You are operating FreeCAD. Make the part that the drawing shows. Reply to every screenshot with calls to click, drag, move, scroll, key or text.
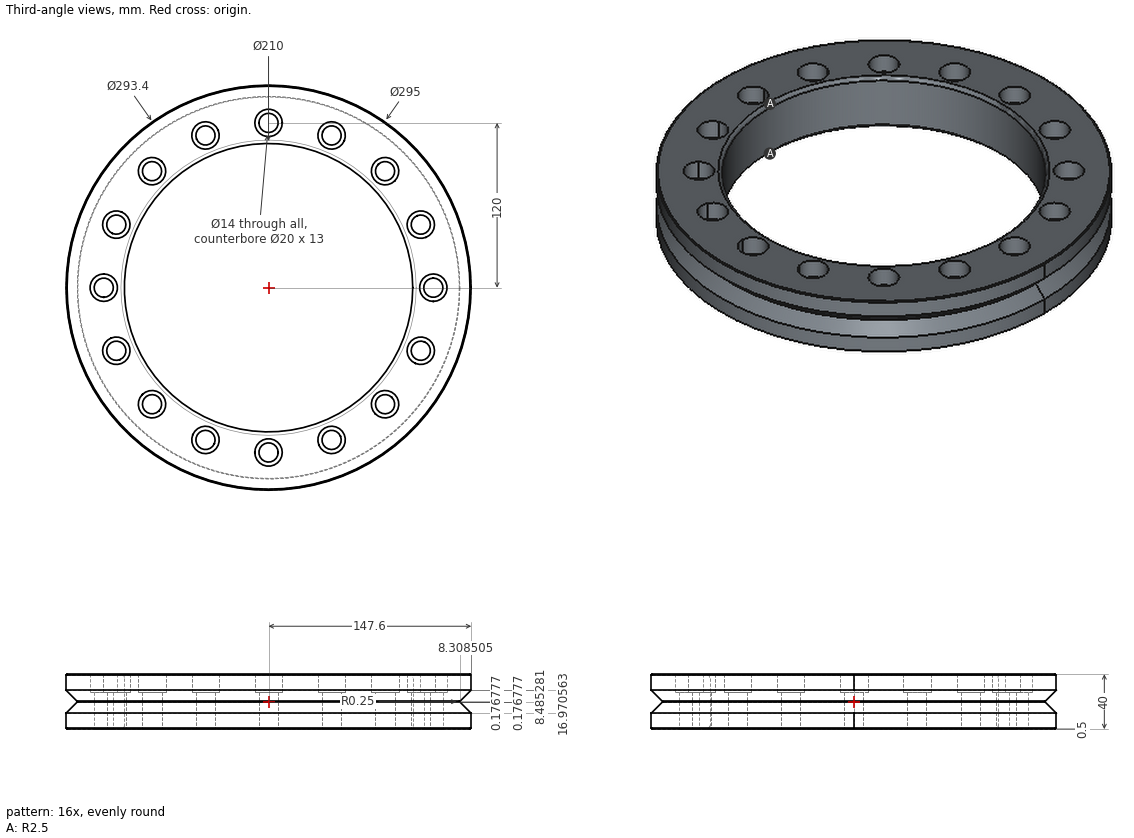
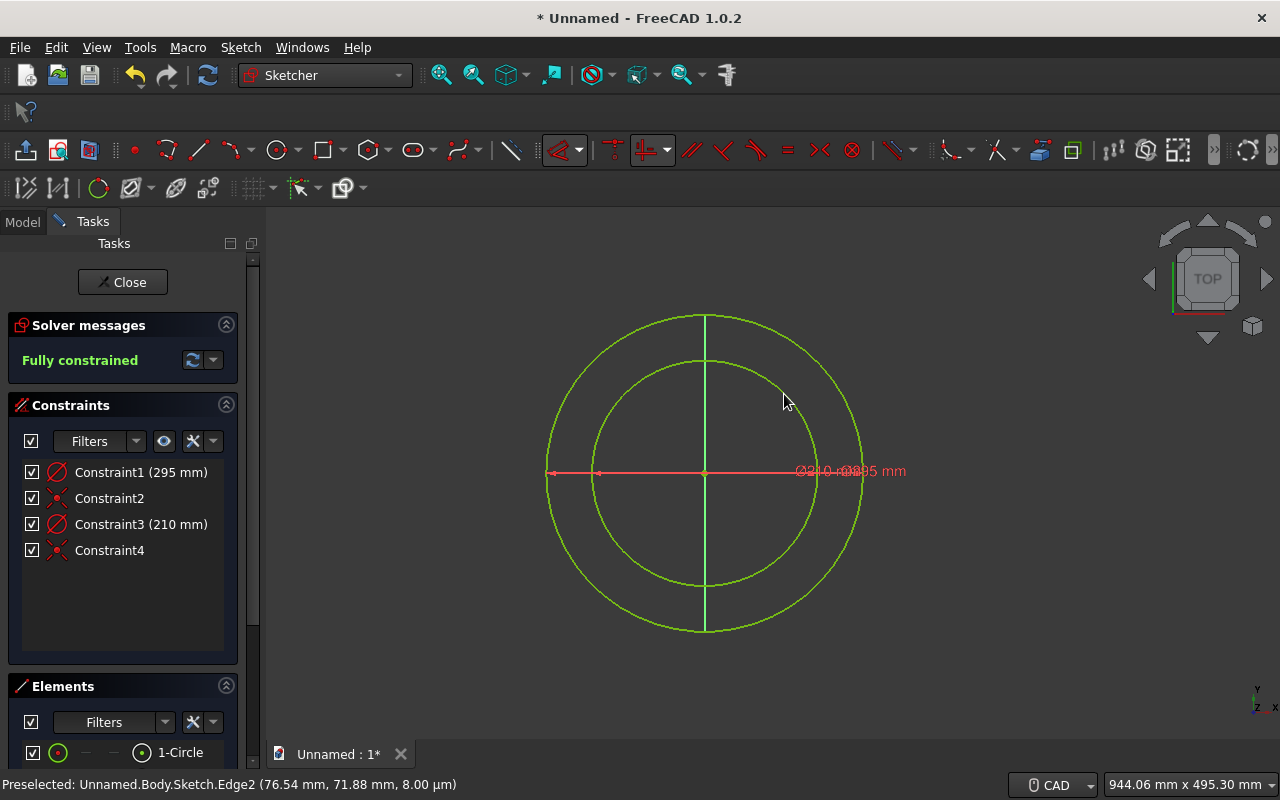
click(123, 282)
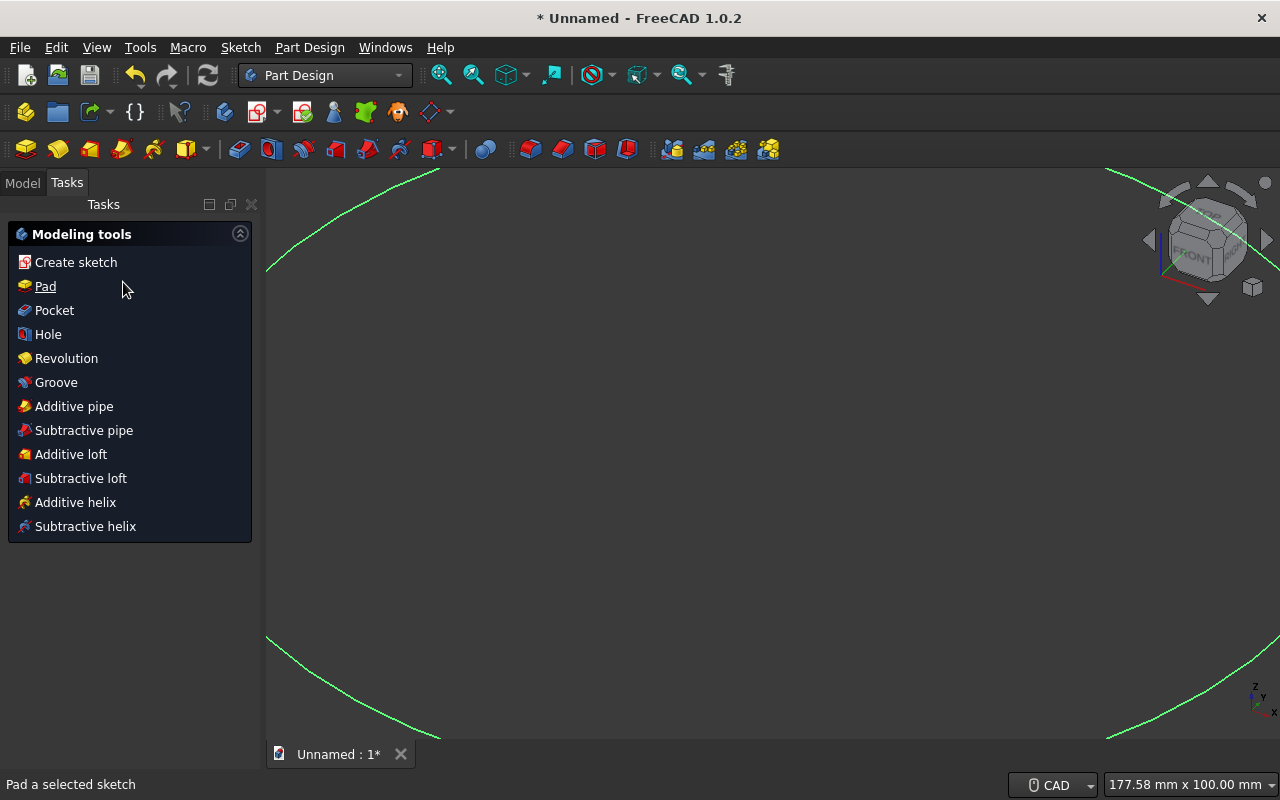
click(26, 150)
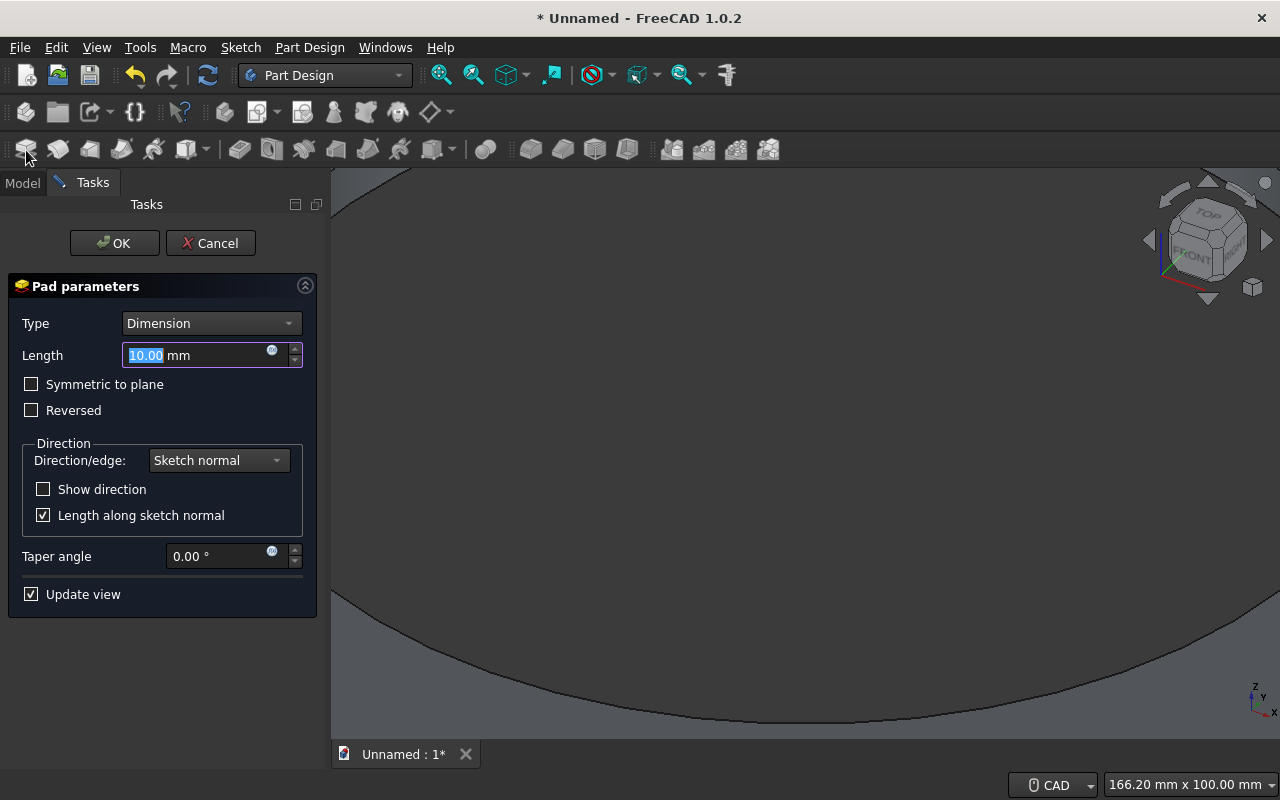
text(40)
key(Tab)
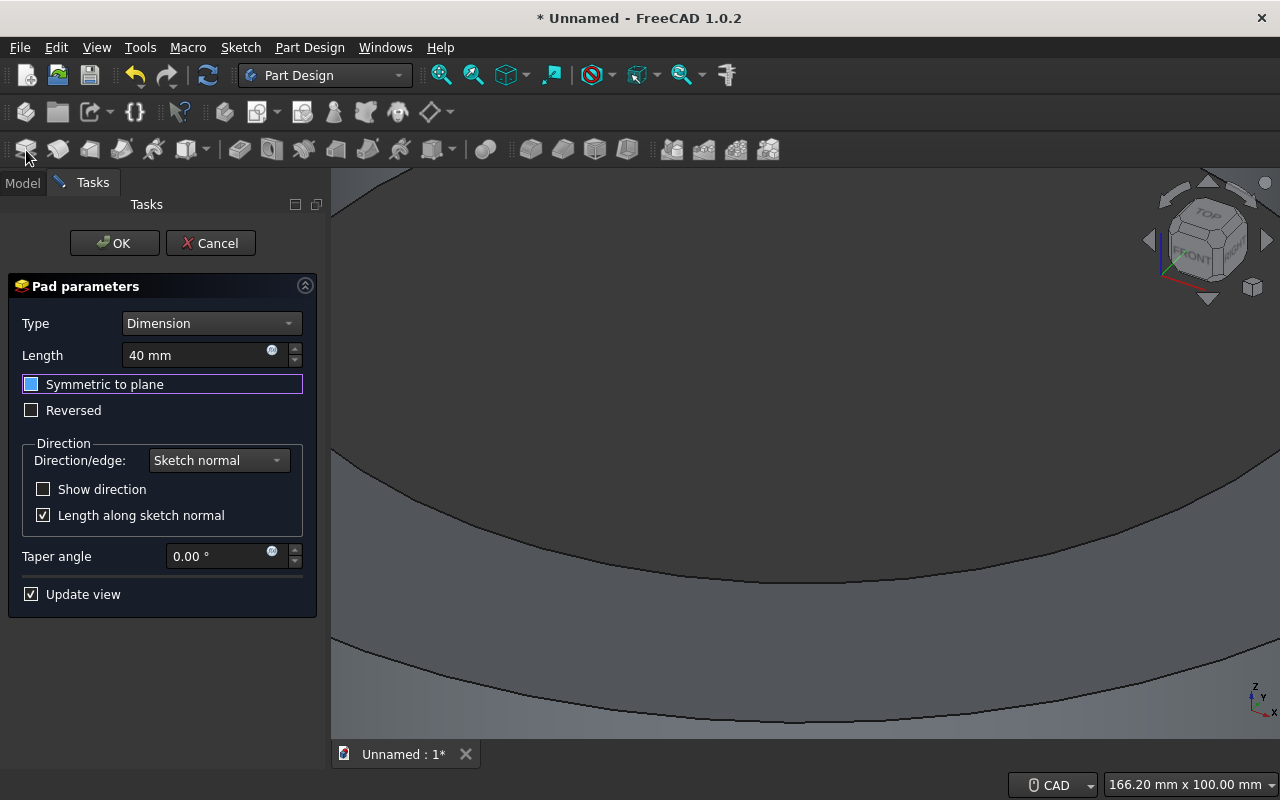
click(30, 384)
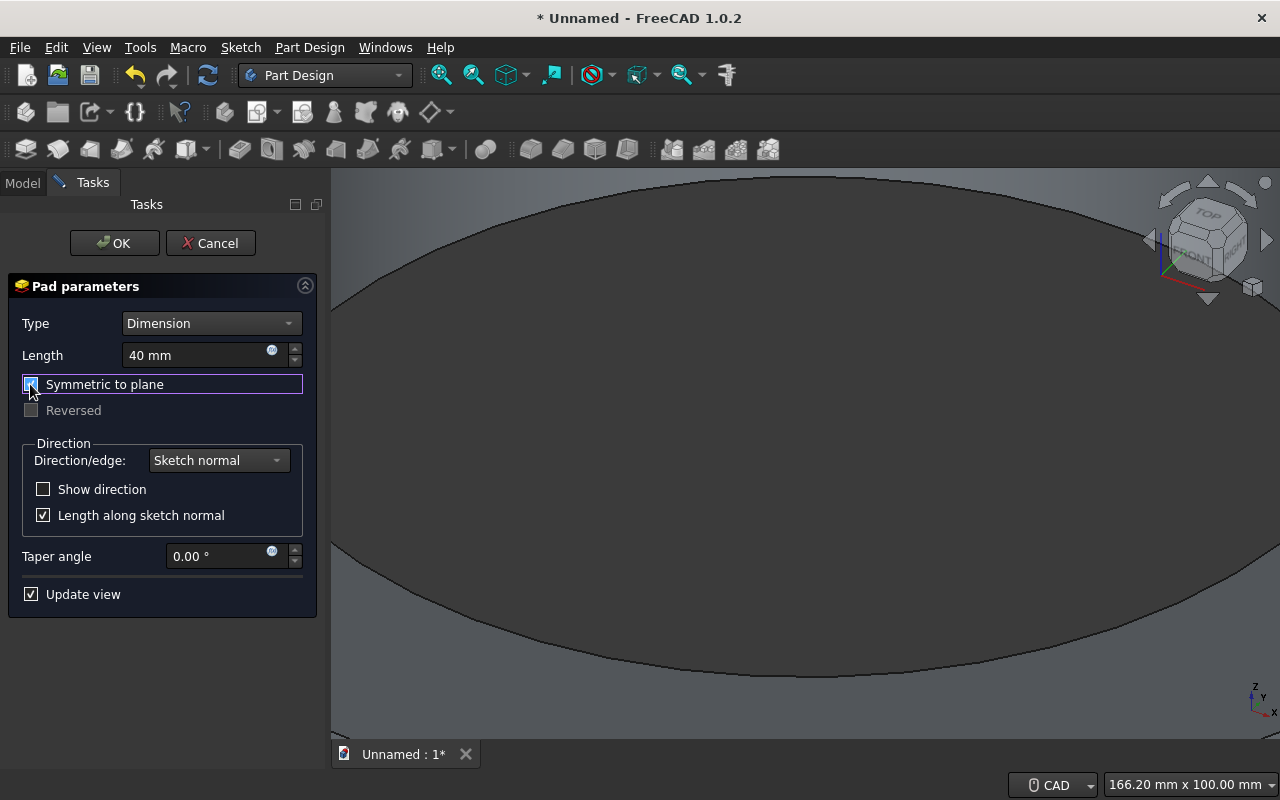
click(115, 243)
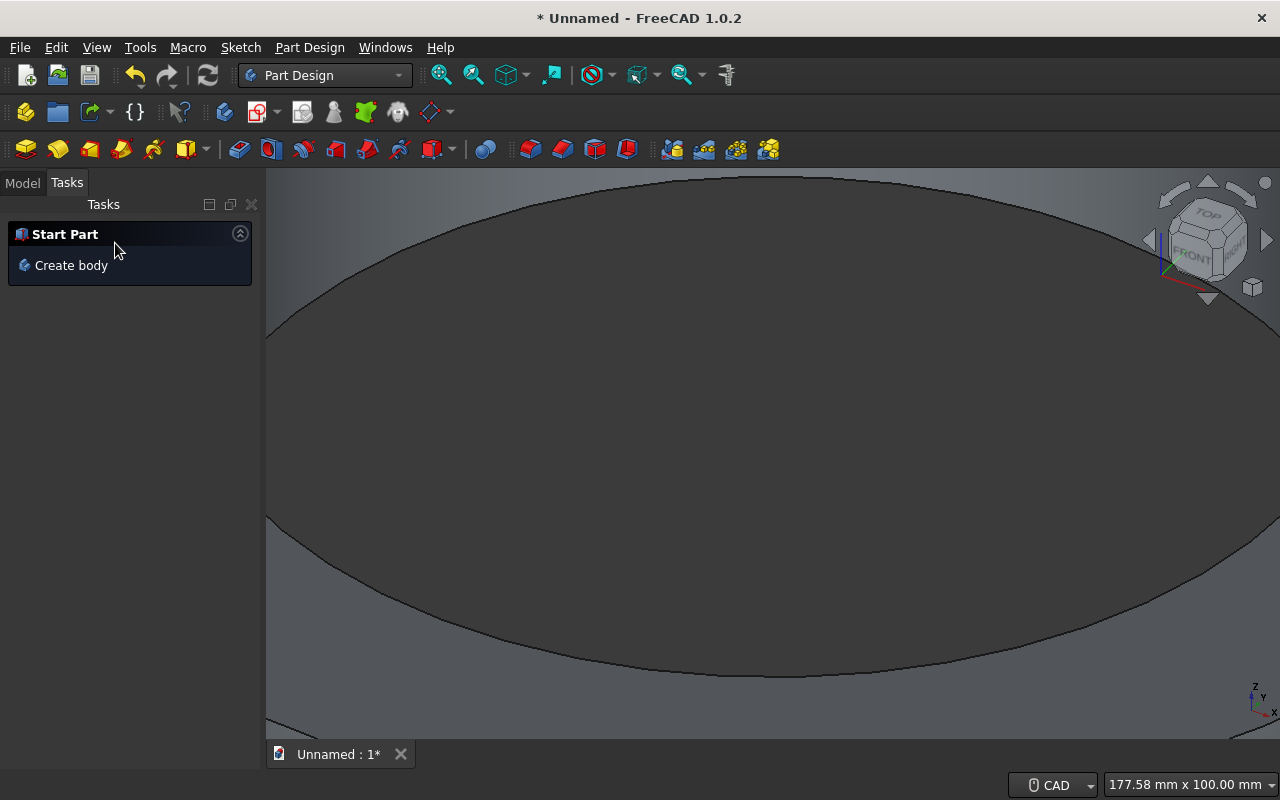
click(442, 76)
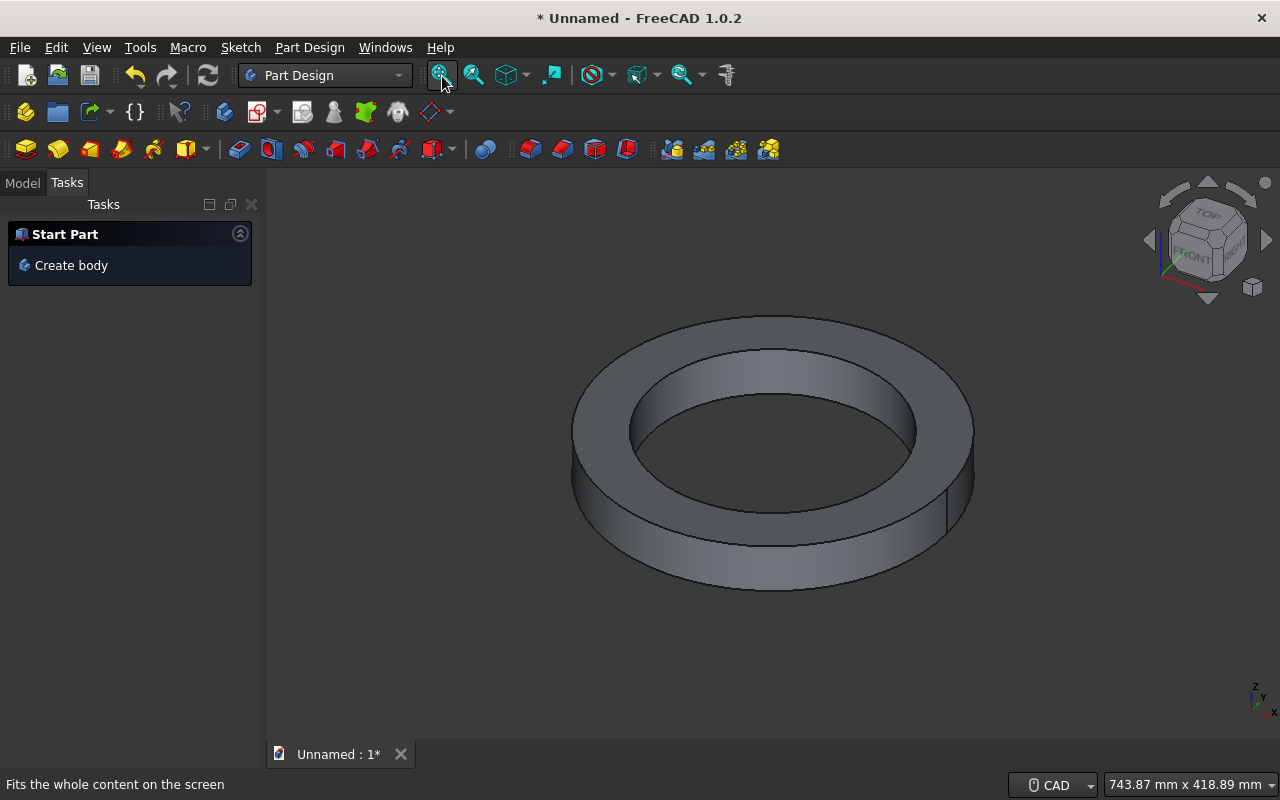
click(922, 480)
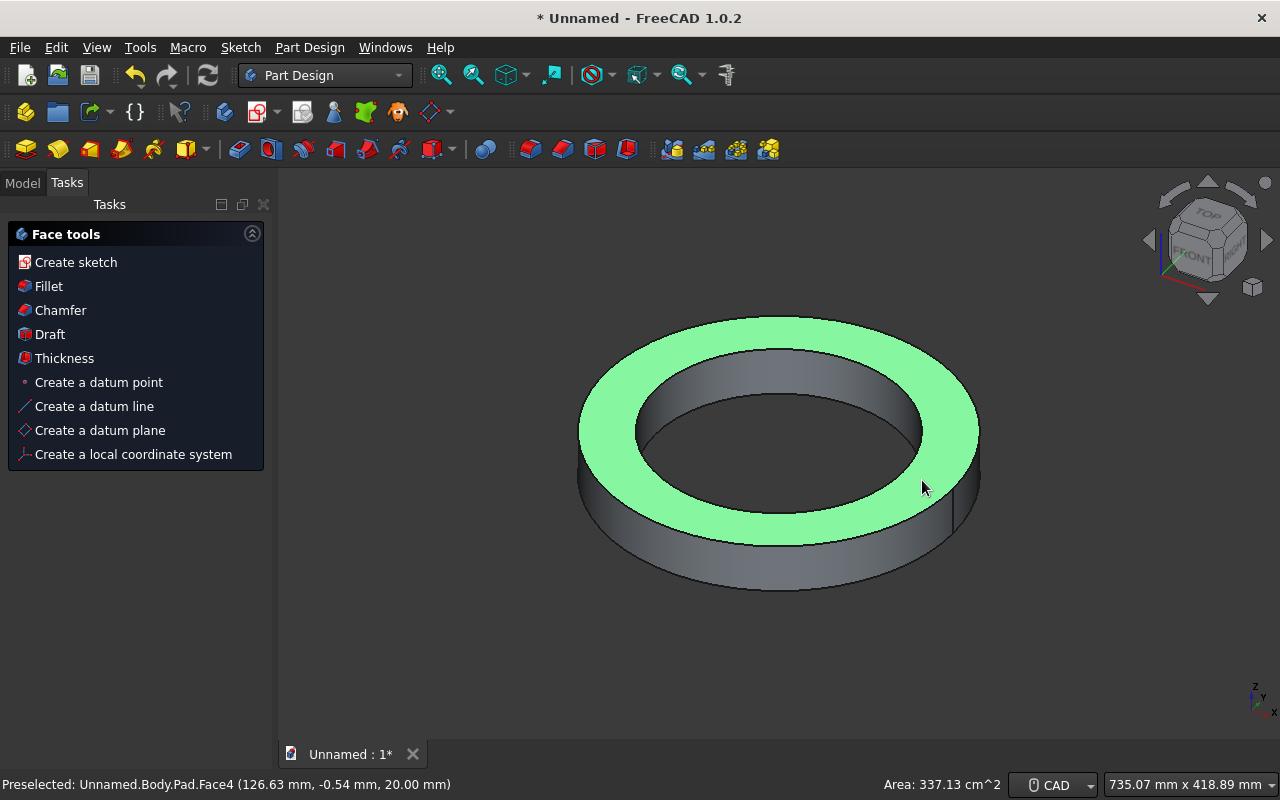
click(258, 112)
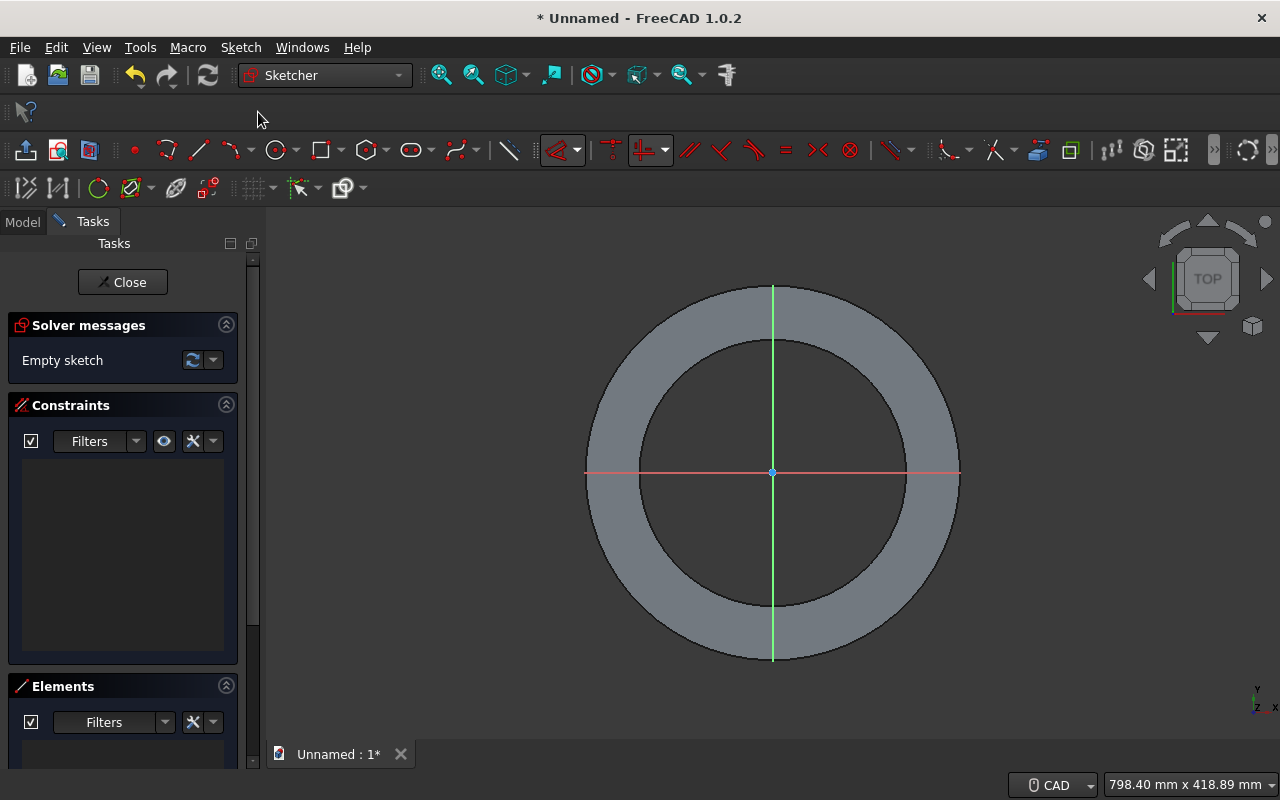
scroll(776, 313, up, 15)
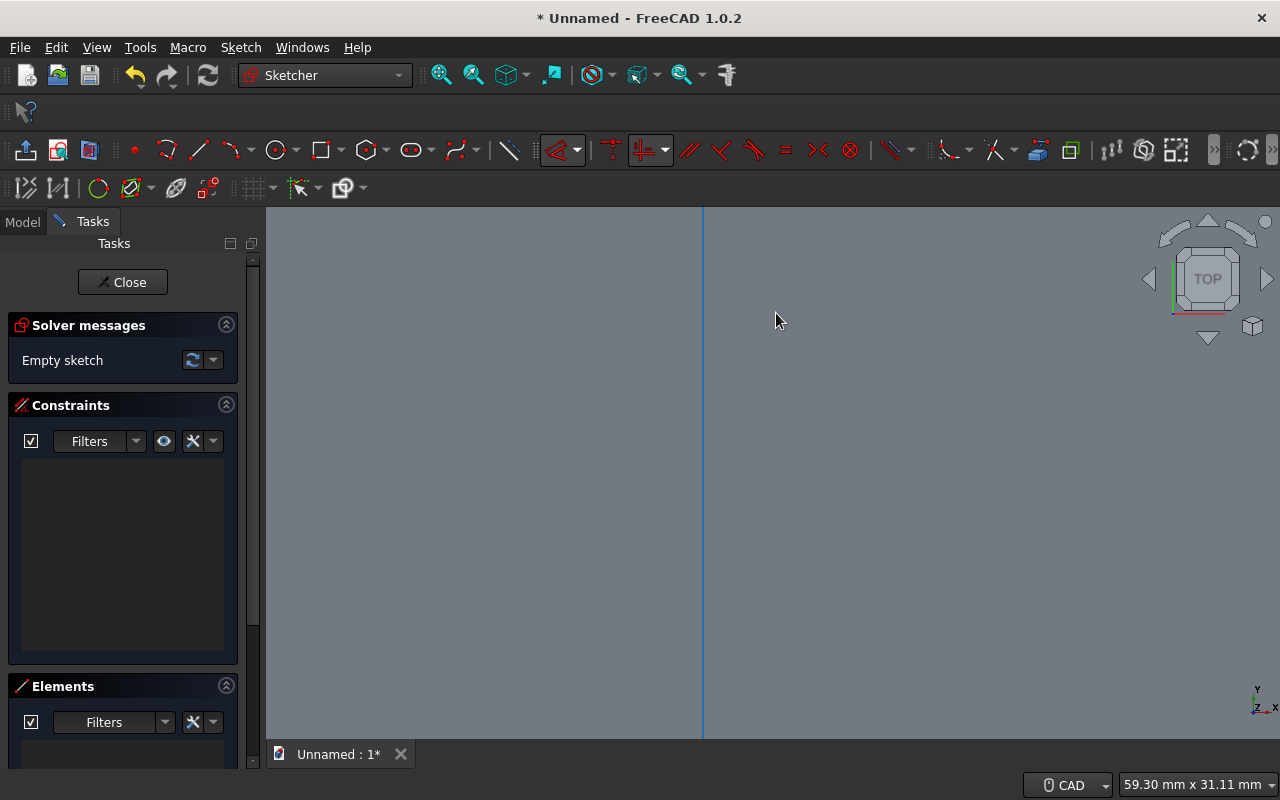
key(g)
key(c)